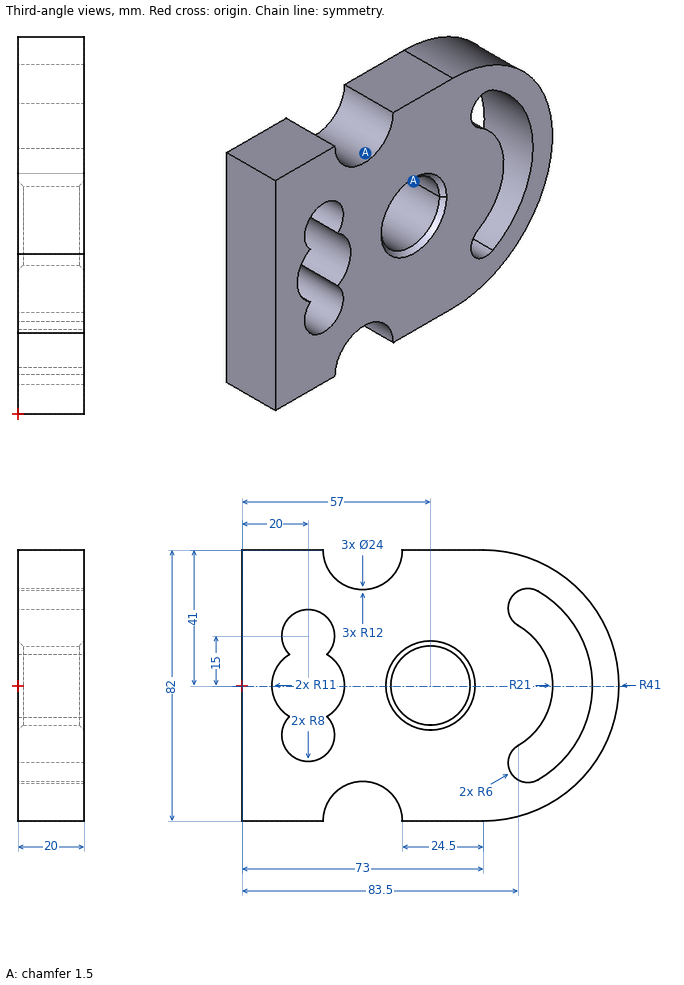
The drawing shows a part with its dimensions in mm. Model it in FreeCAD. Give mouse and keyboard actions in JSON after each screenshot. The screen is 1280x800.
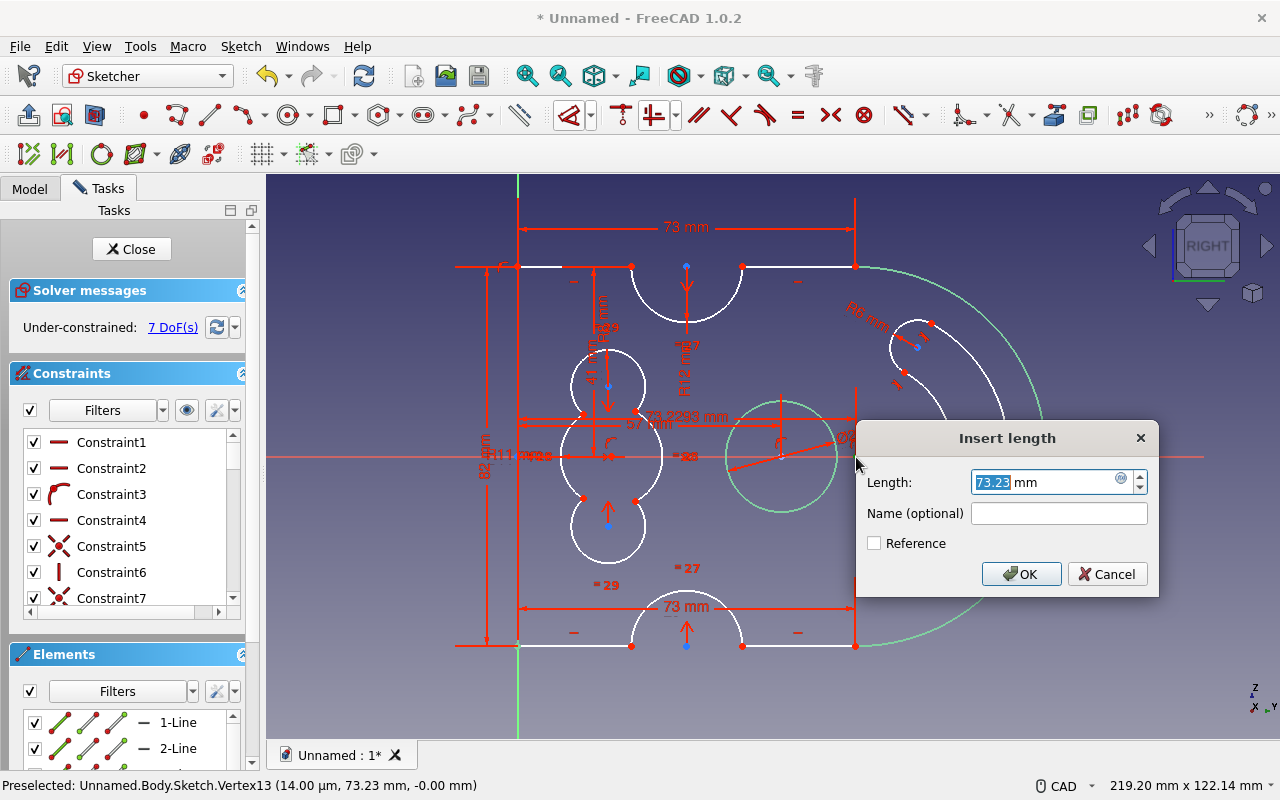
{"action": "type", "text": "73"}
{"action": "key", "text": "Return"}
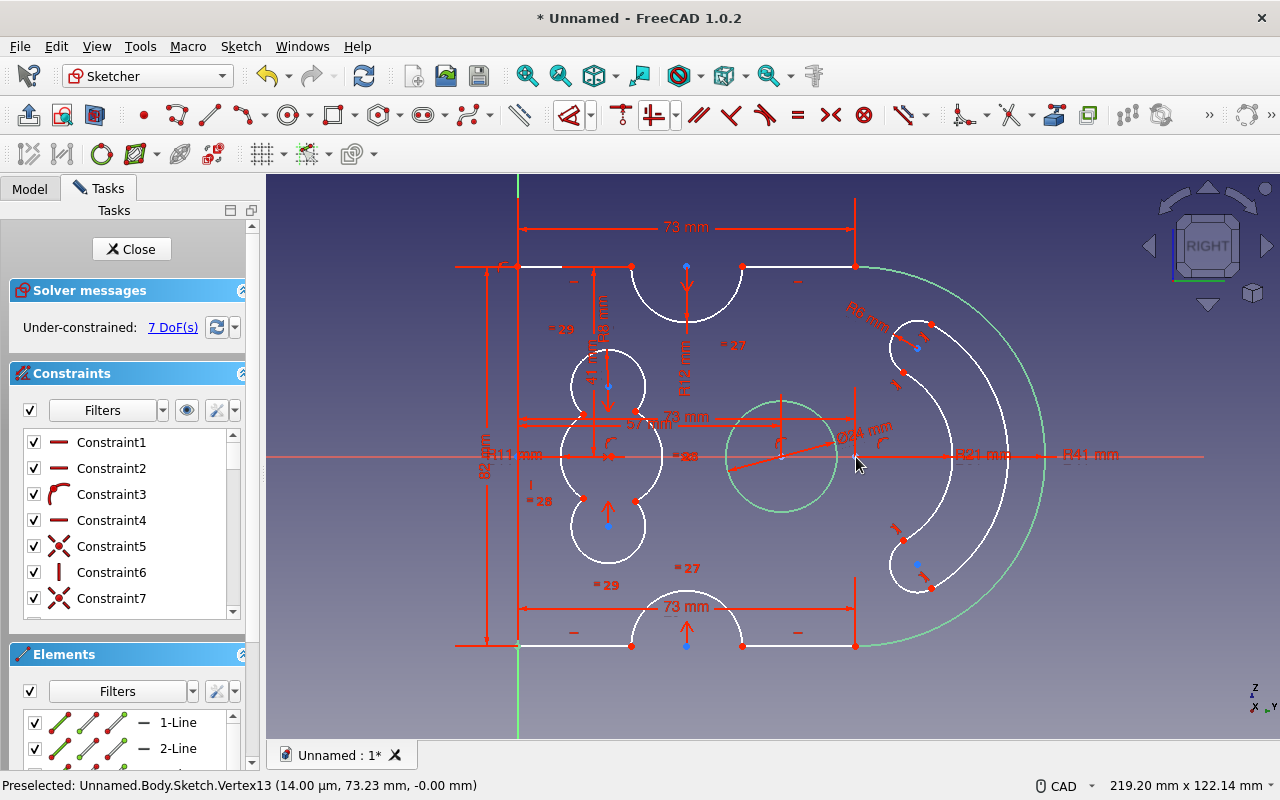
{"action": "left_click", "coordinate": [687, 267]}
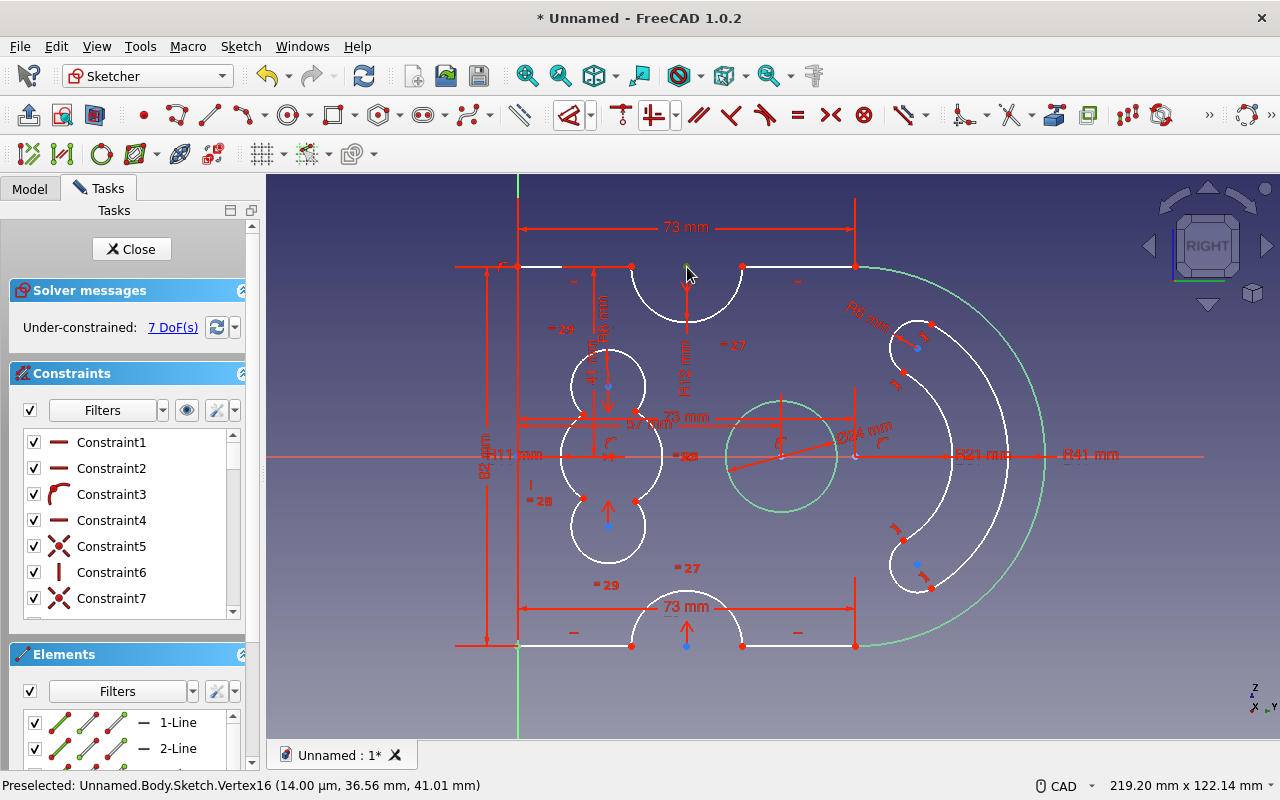
{"action": "key", "text": "i"}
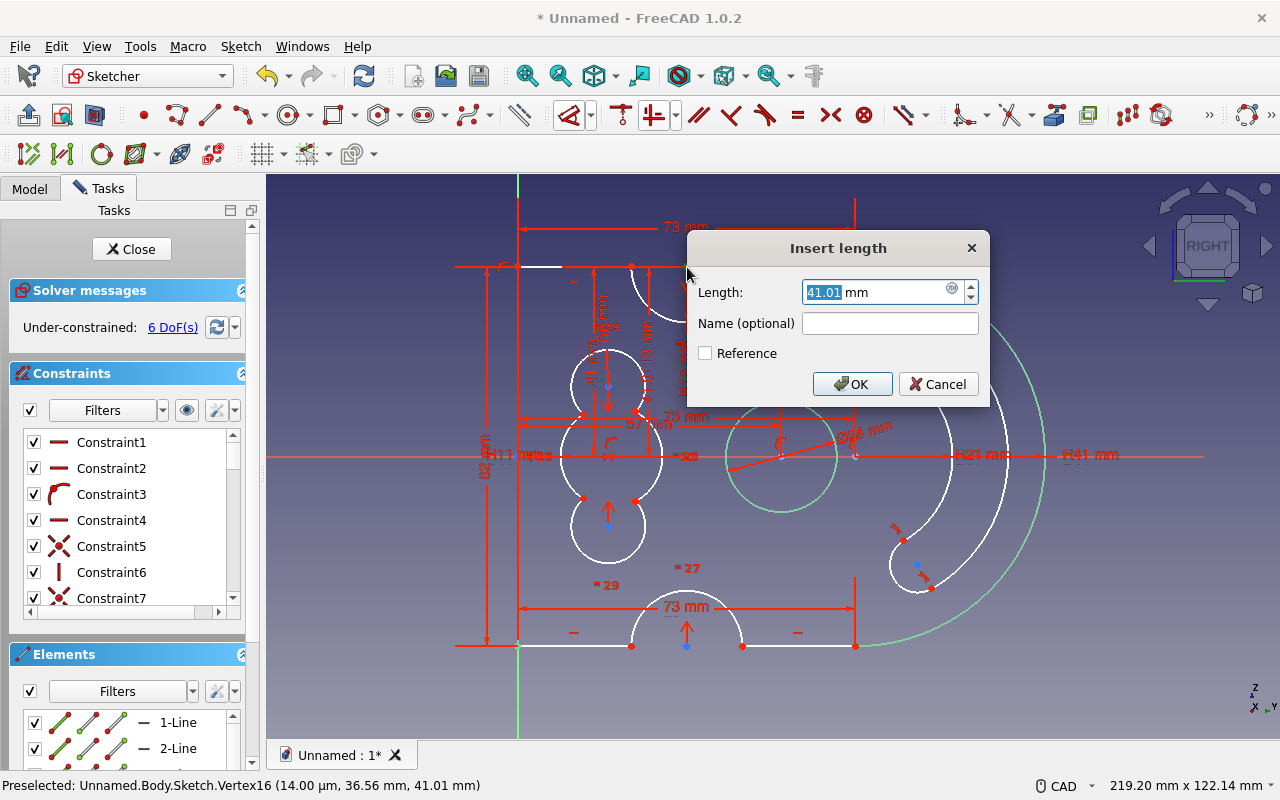
{"action": "type", "text": "41"}
{"action": "key", "text": "Return"}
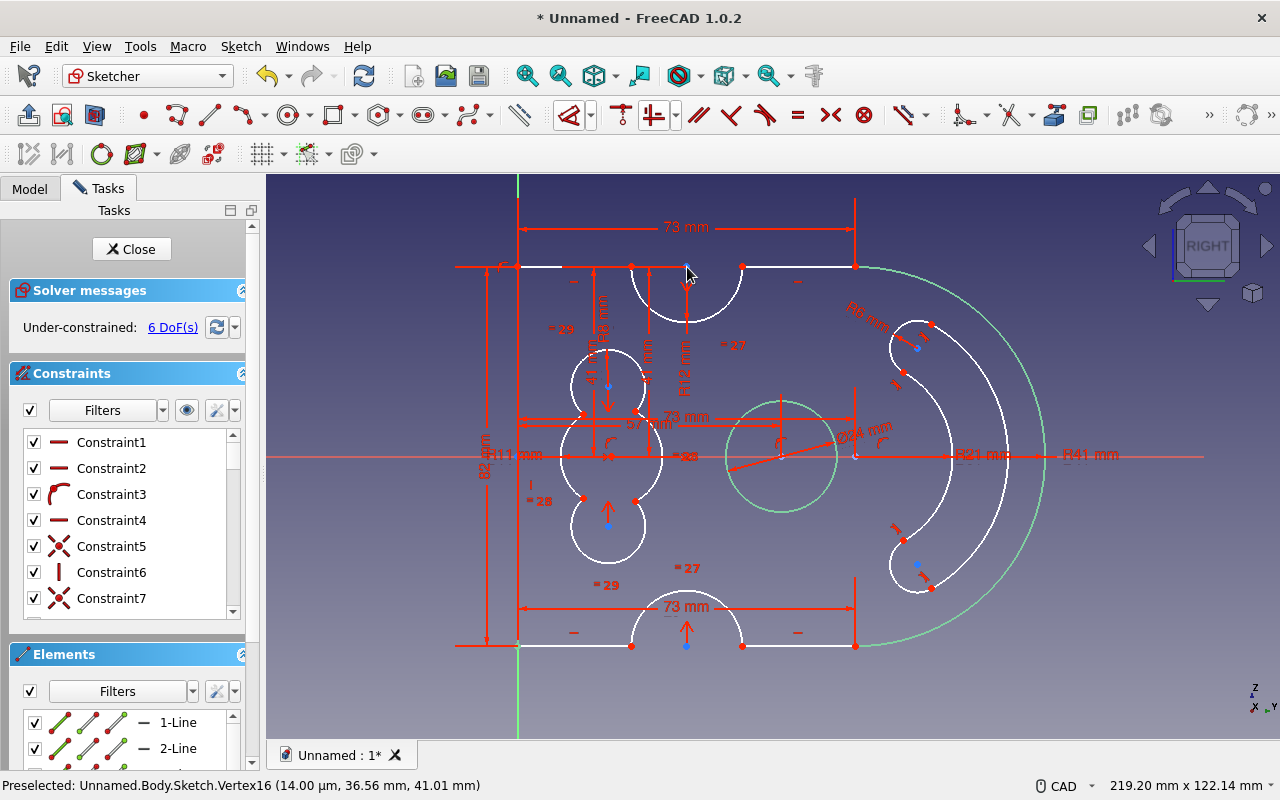
{"action": "left_click", "coordinate": [611, 457]}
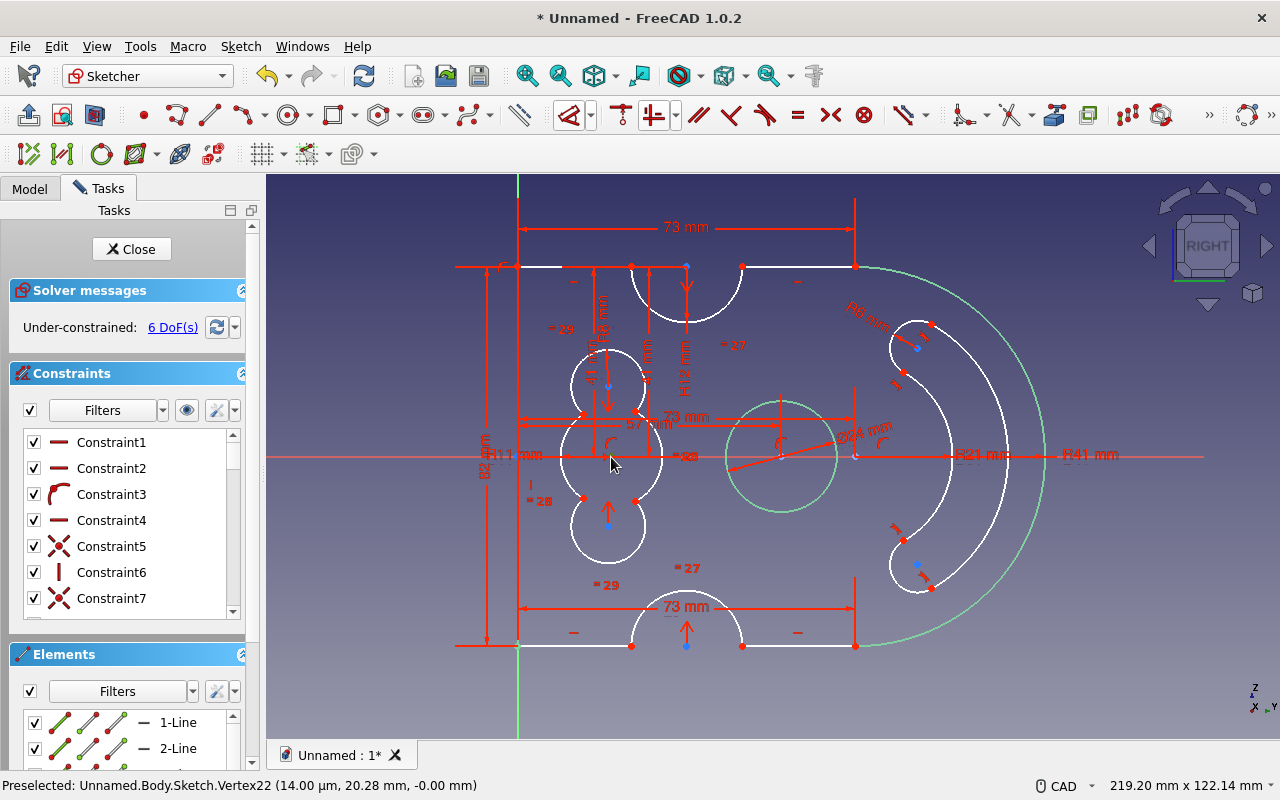
{"action": "key", "text": "l"}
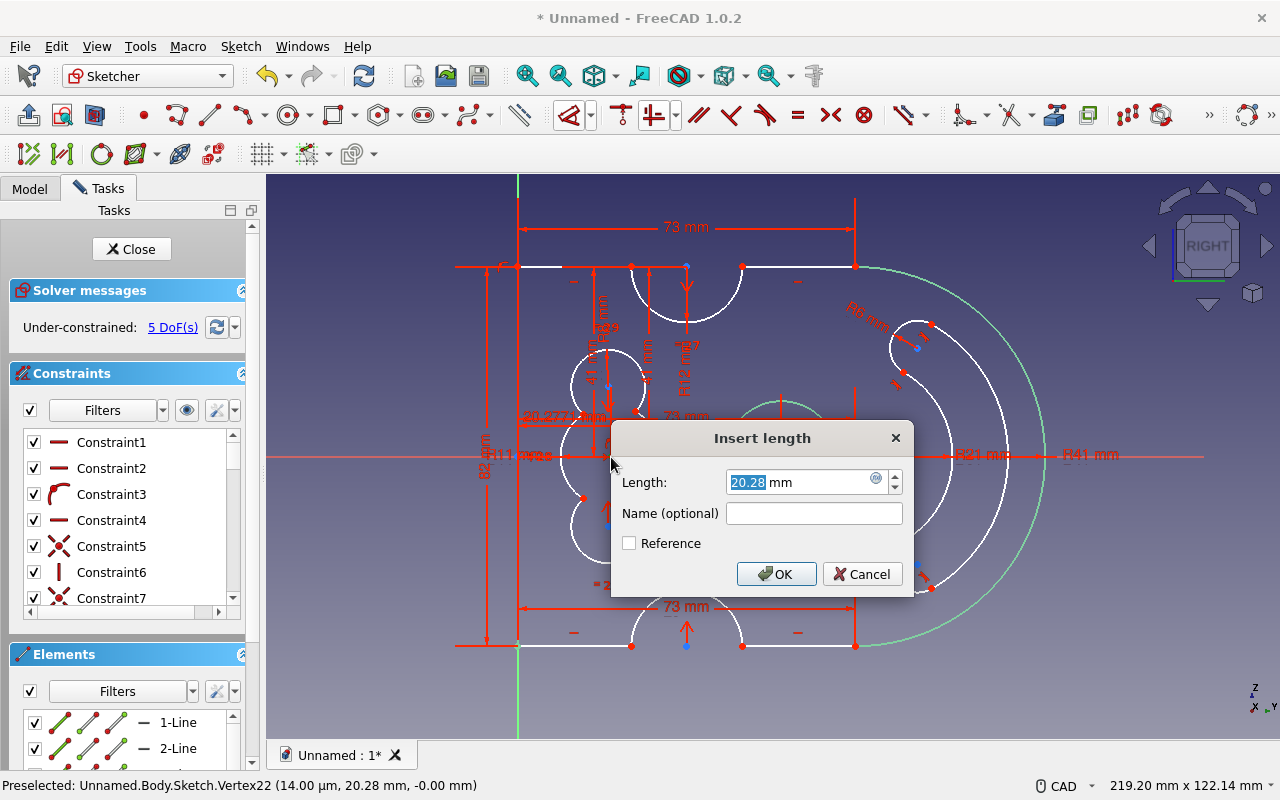
{"action": "type", "text": "20"}
{"action": "key", "text": "Return"}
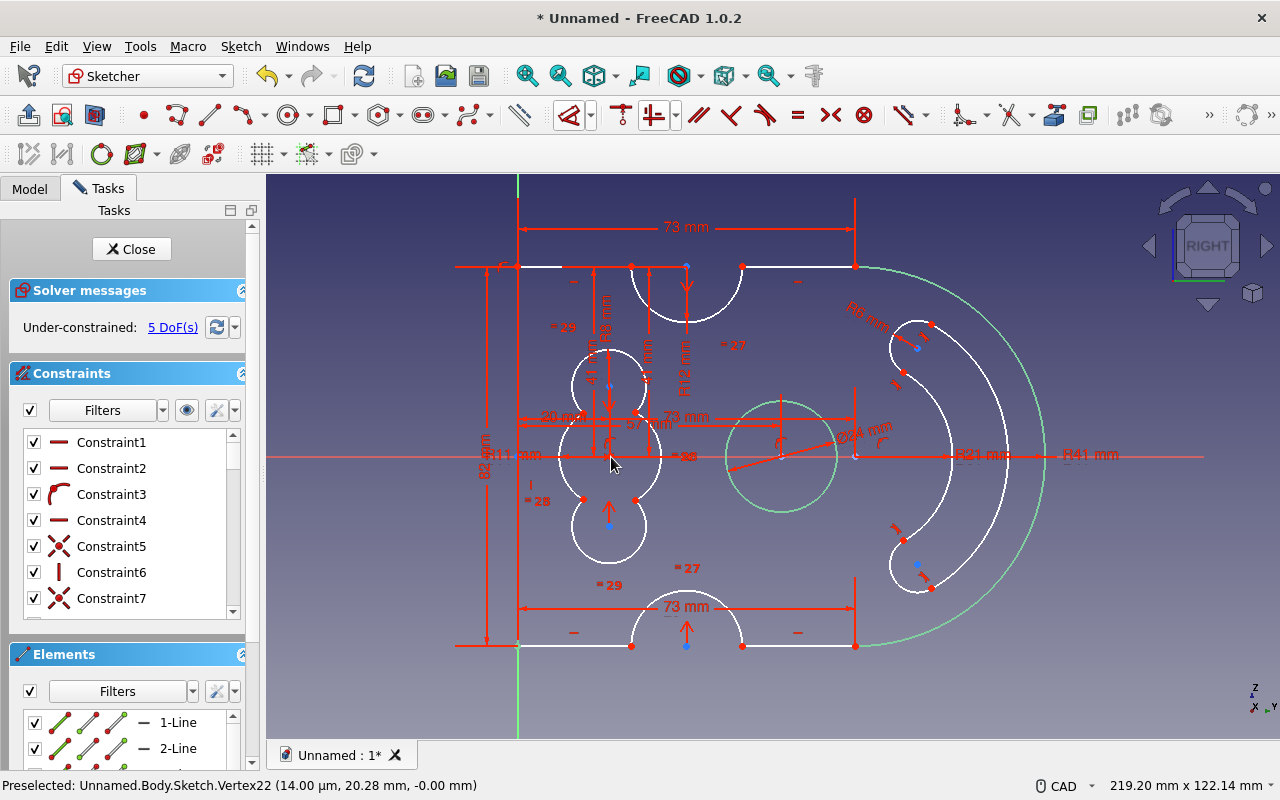
{"action": "left_click", "coordinate": [609, 387]}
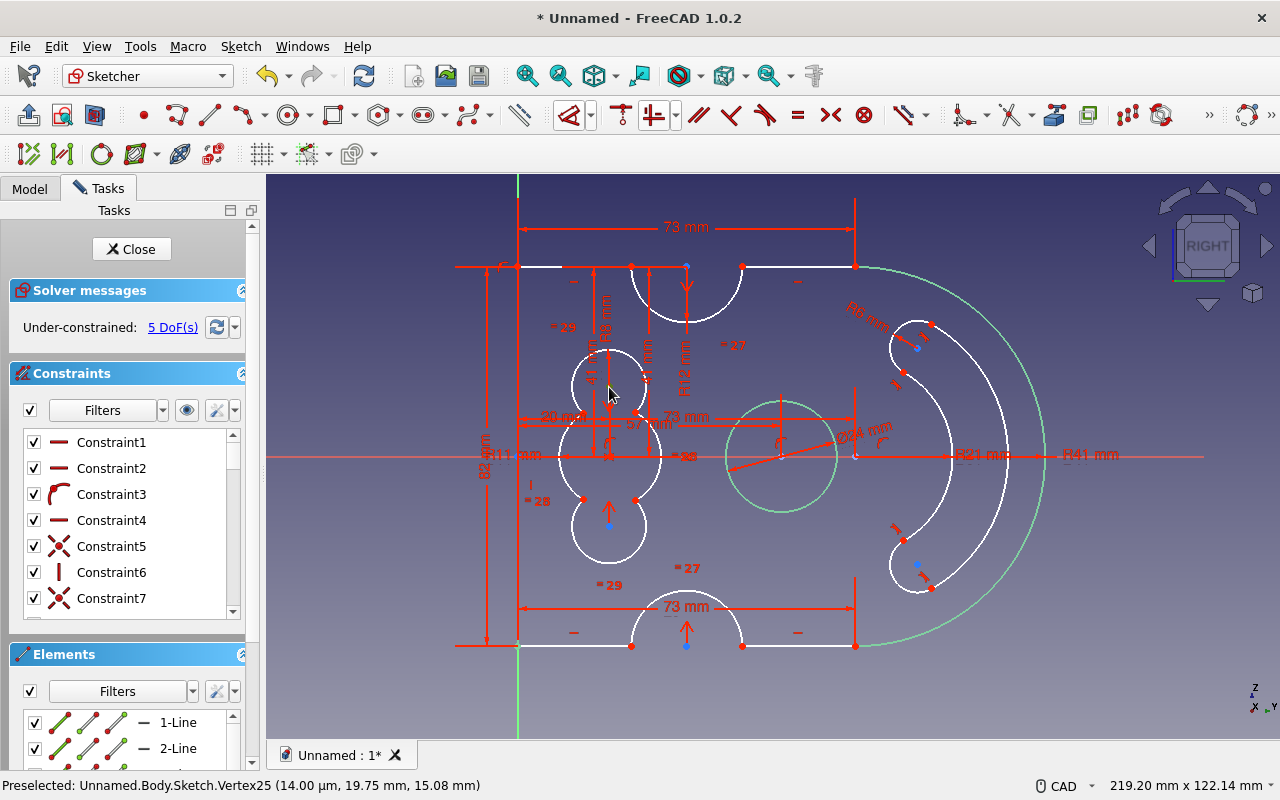
{"action": "key", "text": "l"}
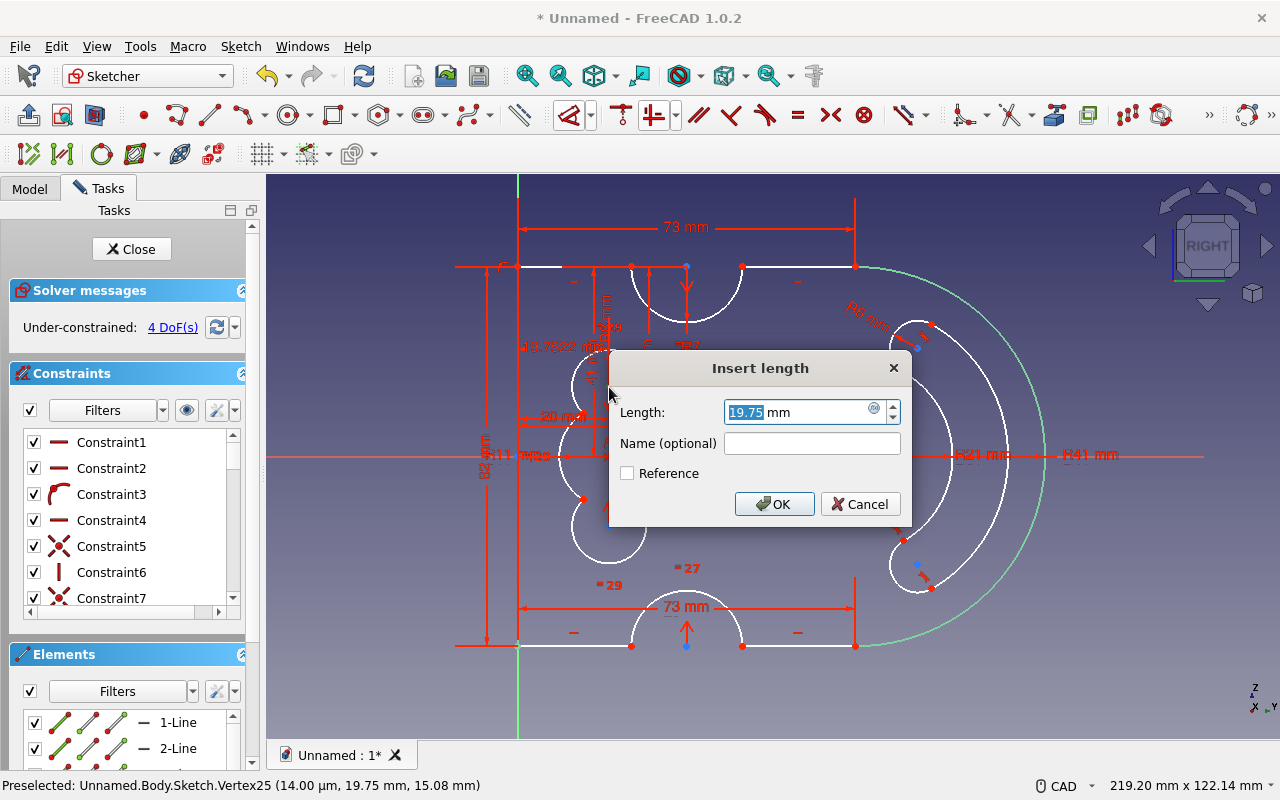
{"action": "type", "text": "20"}
{"action": "key", "text": "Return"}